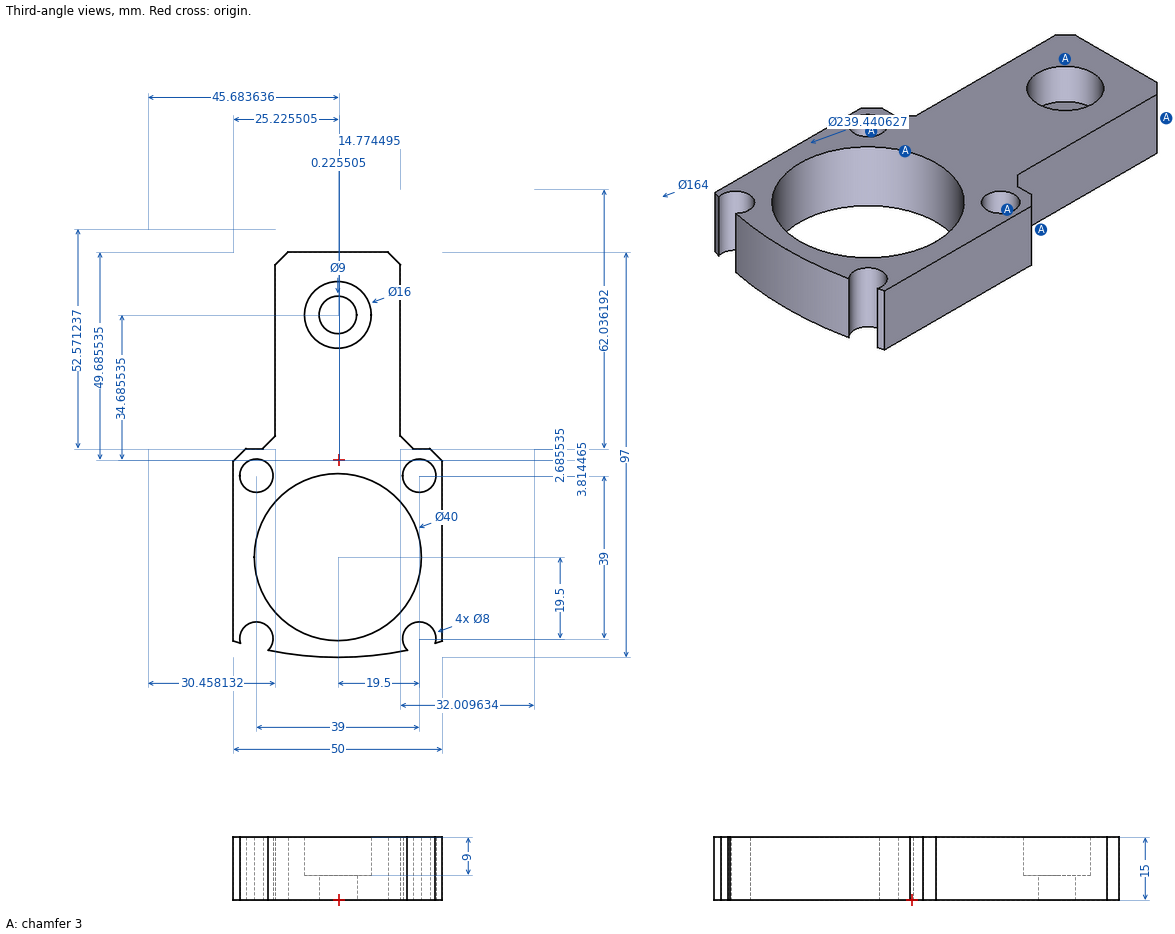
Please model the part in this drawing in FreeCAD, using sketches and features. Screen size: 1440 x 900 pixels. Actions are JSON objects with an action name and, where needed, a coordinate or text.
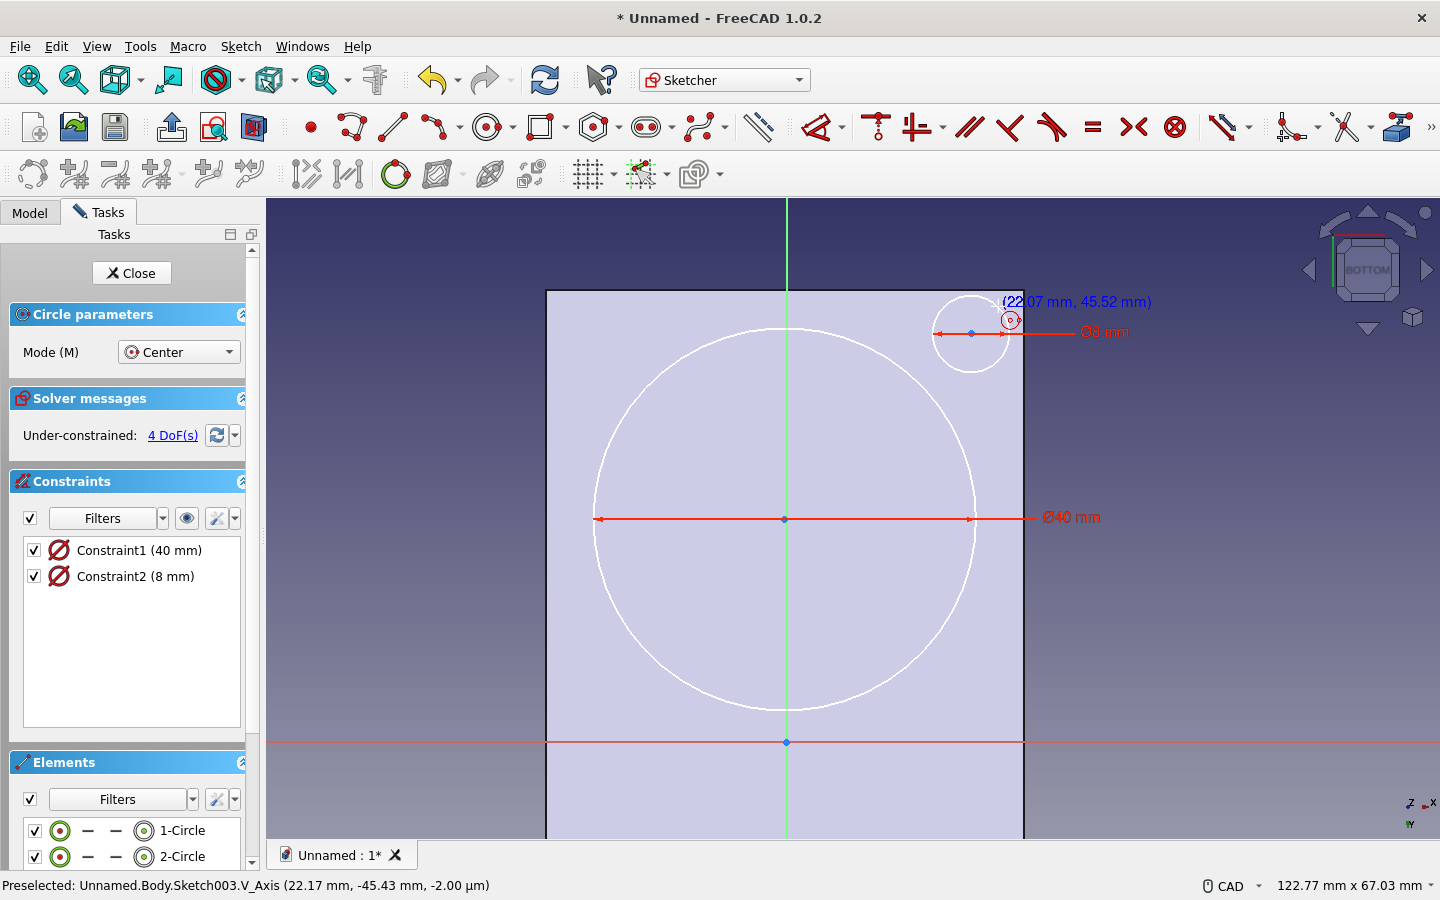
{"action": "left_click", "coordinate": [971, 706]}
{"action": "mouse_move", "coordinate": [998, 679]}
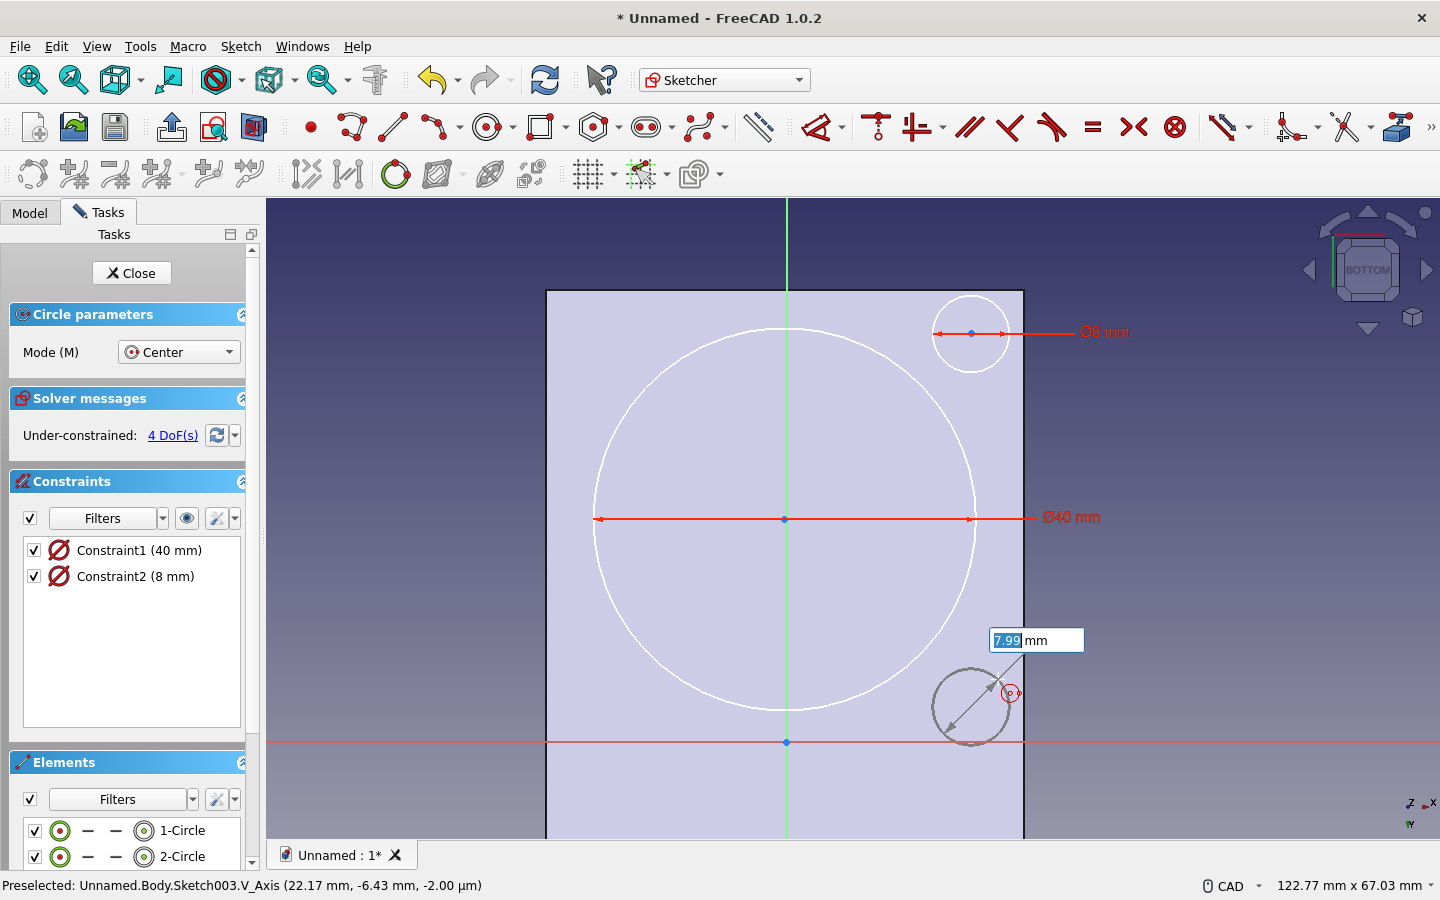
{"action": "type", "text": "8"}
{"action": "key", "text": "Return"}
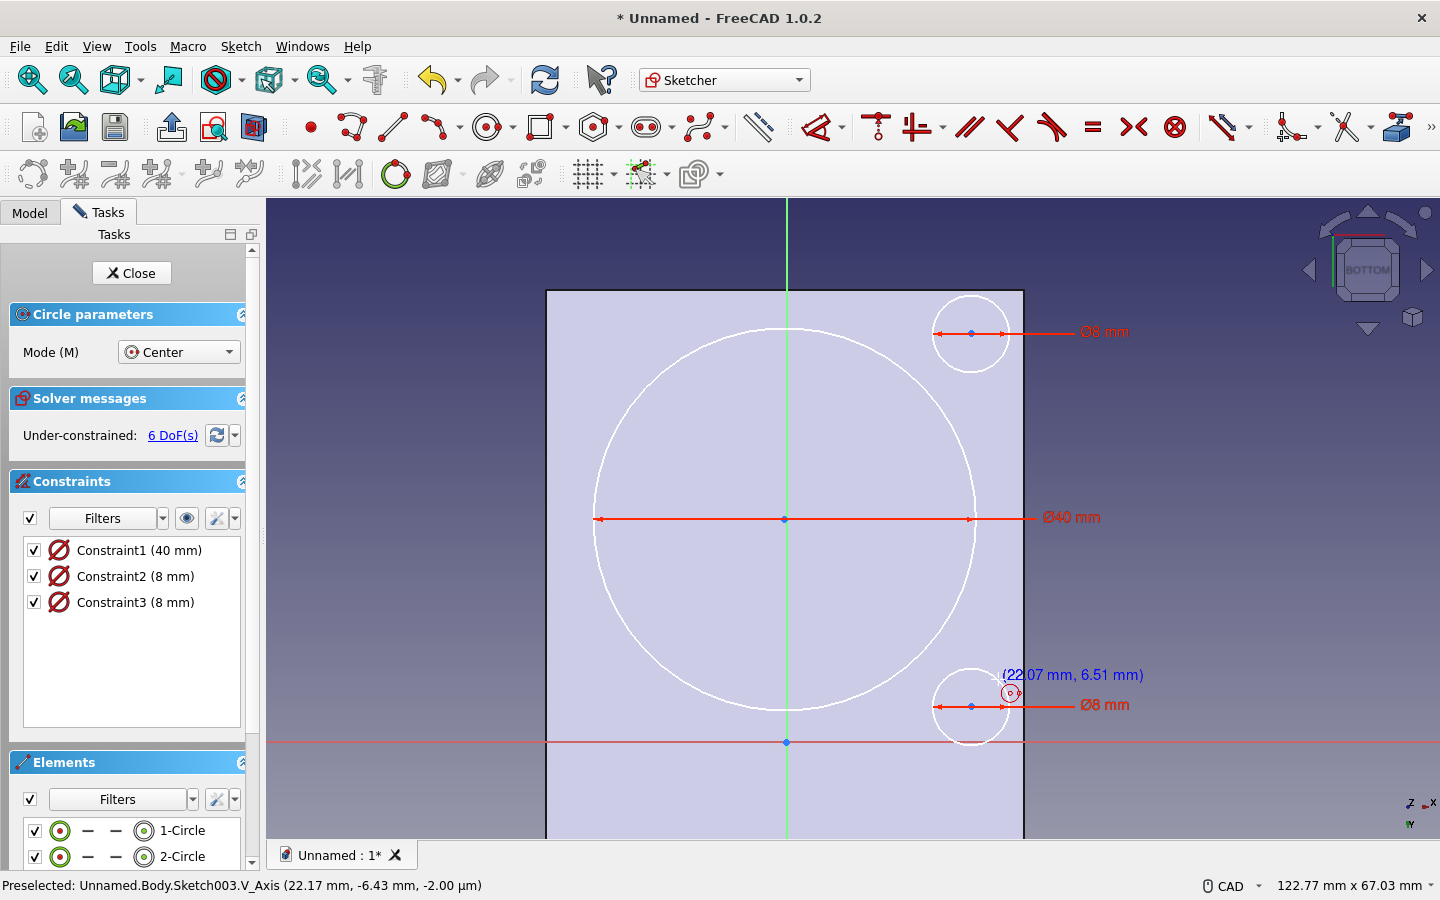
{"action": "left_click", "coordinate": [598, 706]}
{"action": "mouse_move", "coordinate": [625, 679]}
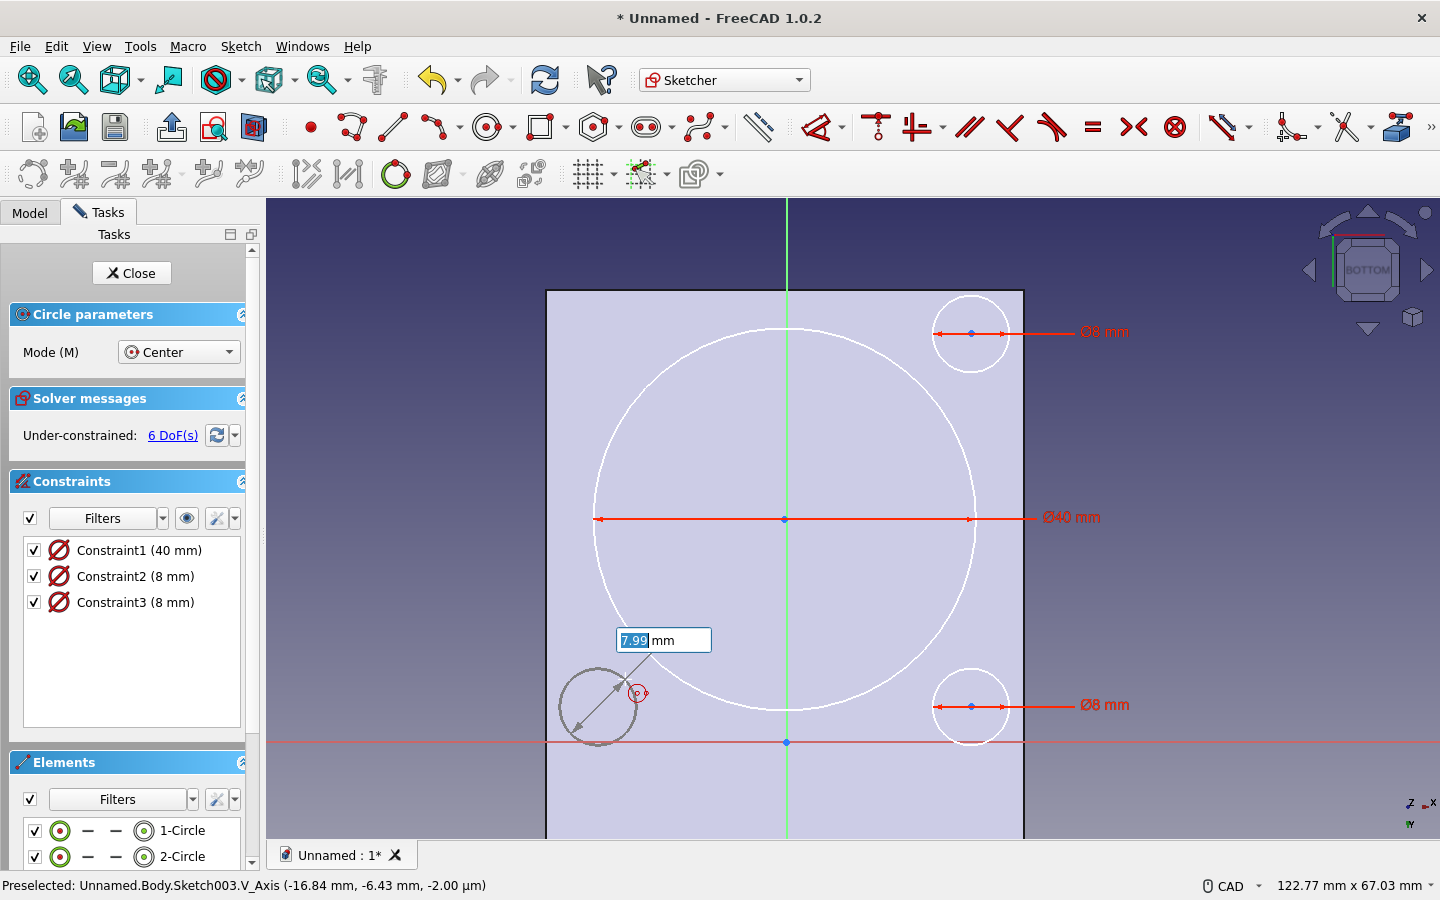
{"action": "type", "text": "8"}
{"action": "key", "text": "Return"}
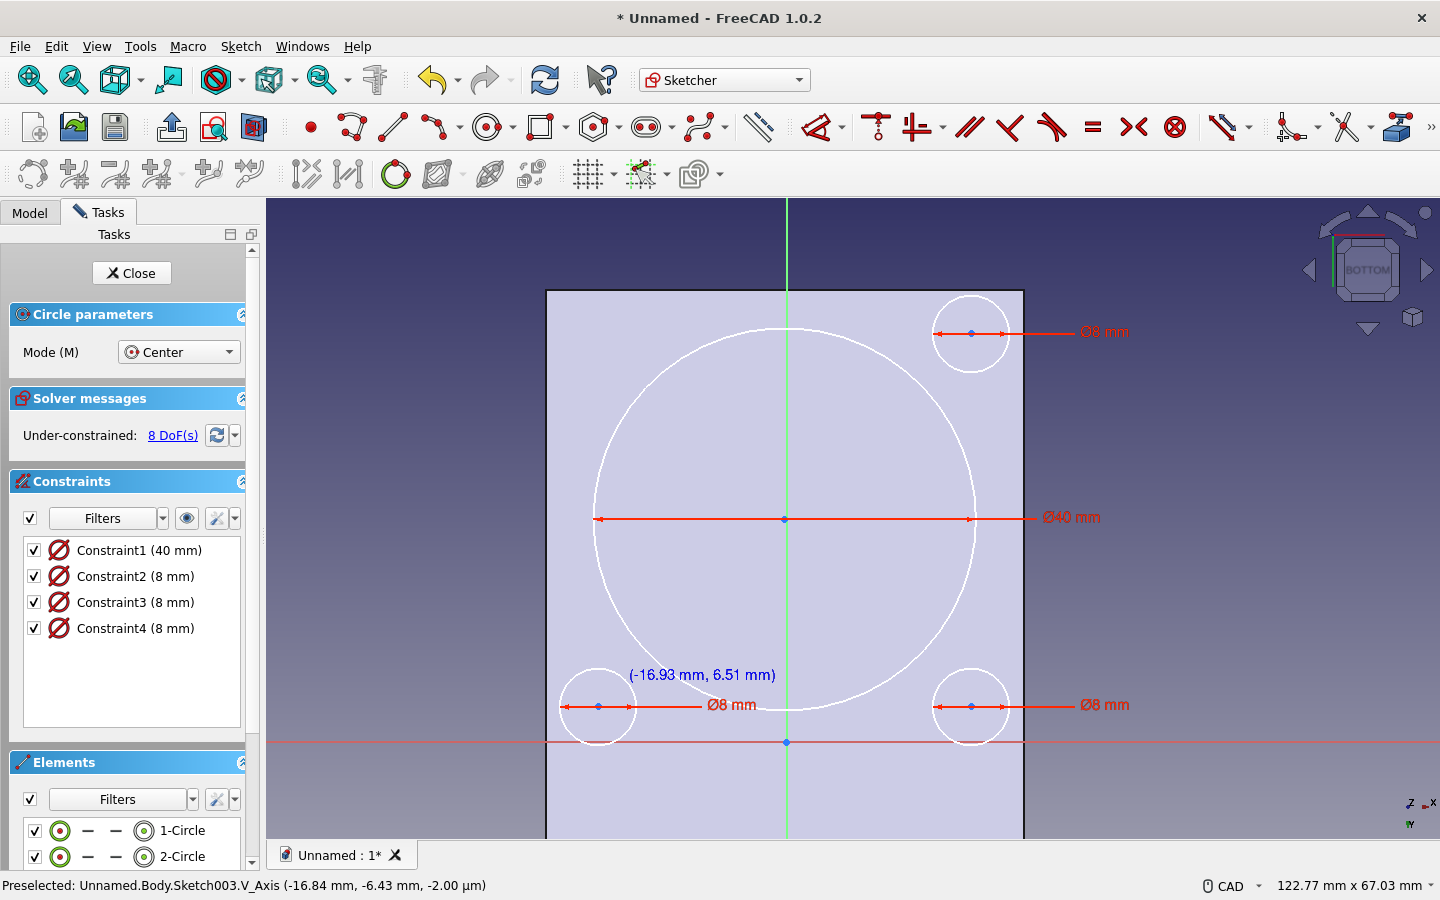
{"action": "left_click", "coordinate": [598, 333]}
{"action": "mouse_move", "coordinate": [625, 306]}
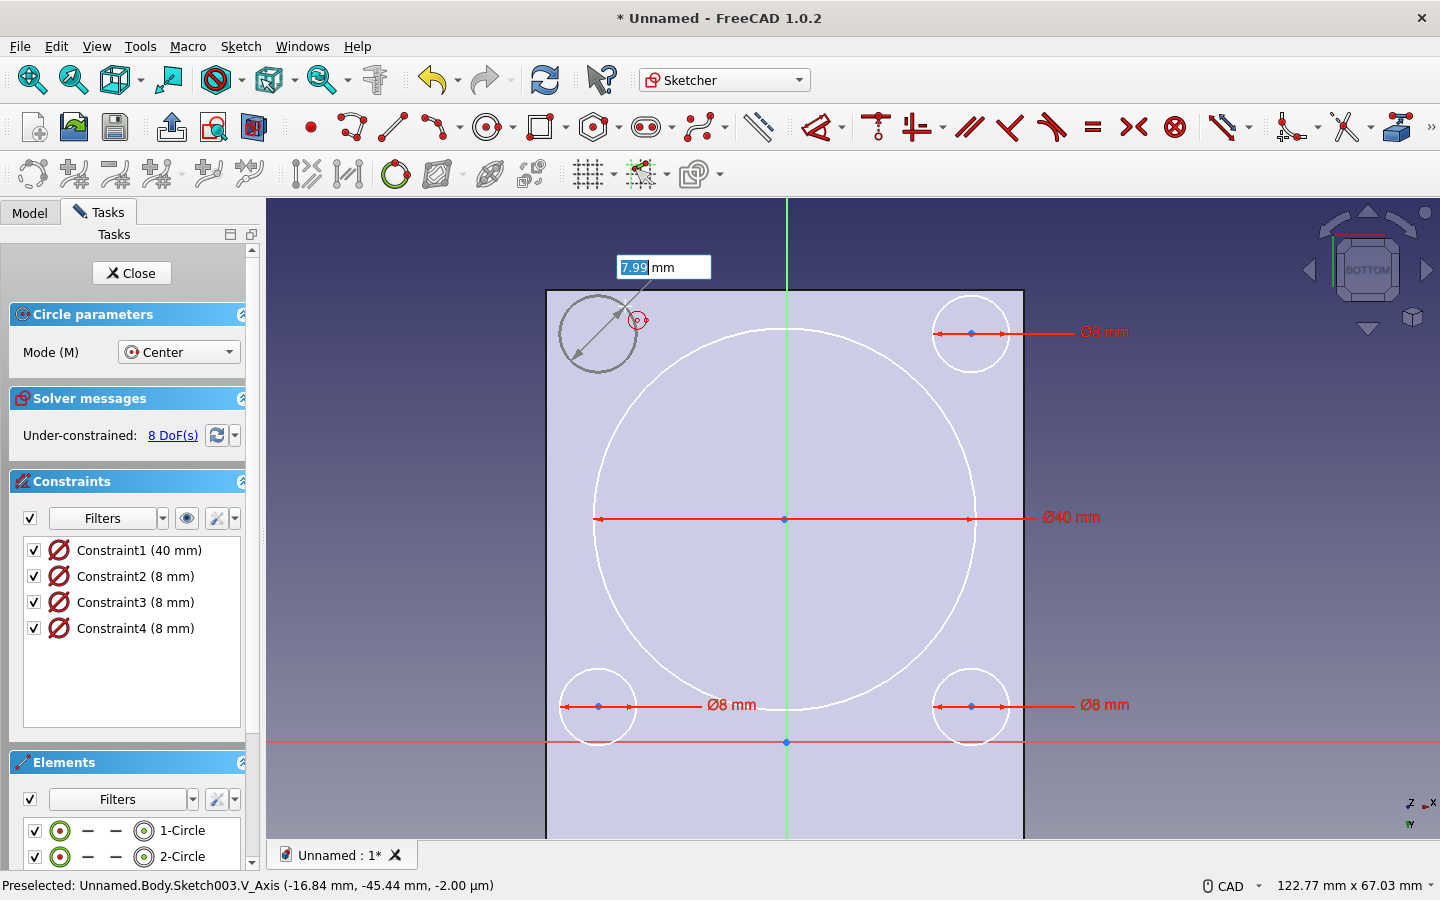
{"action": "type", "text": "8"}
{"action": "key", "text": "Return"}
{"action": "key", "text": "Escape"}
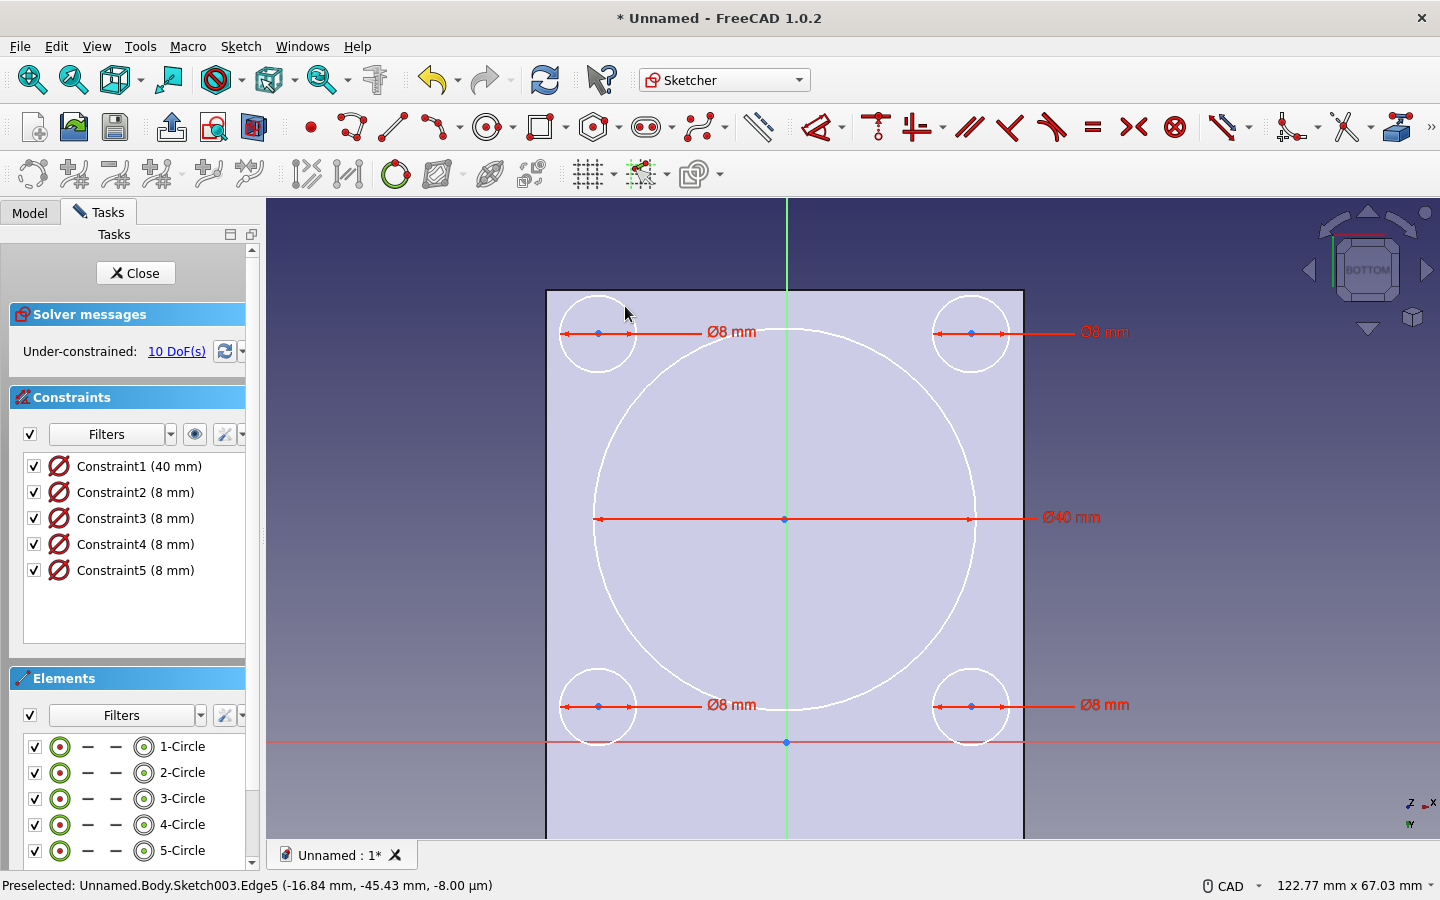
{"action": "left_click", "coordinate": [971, 334]}